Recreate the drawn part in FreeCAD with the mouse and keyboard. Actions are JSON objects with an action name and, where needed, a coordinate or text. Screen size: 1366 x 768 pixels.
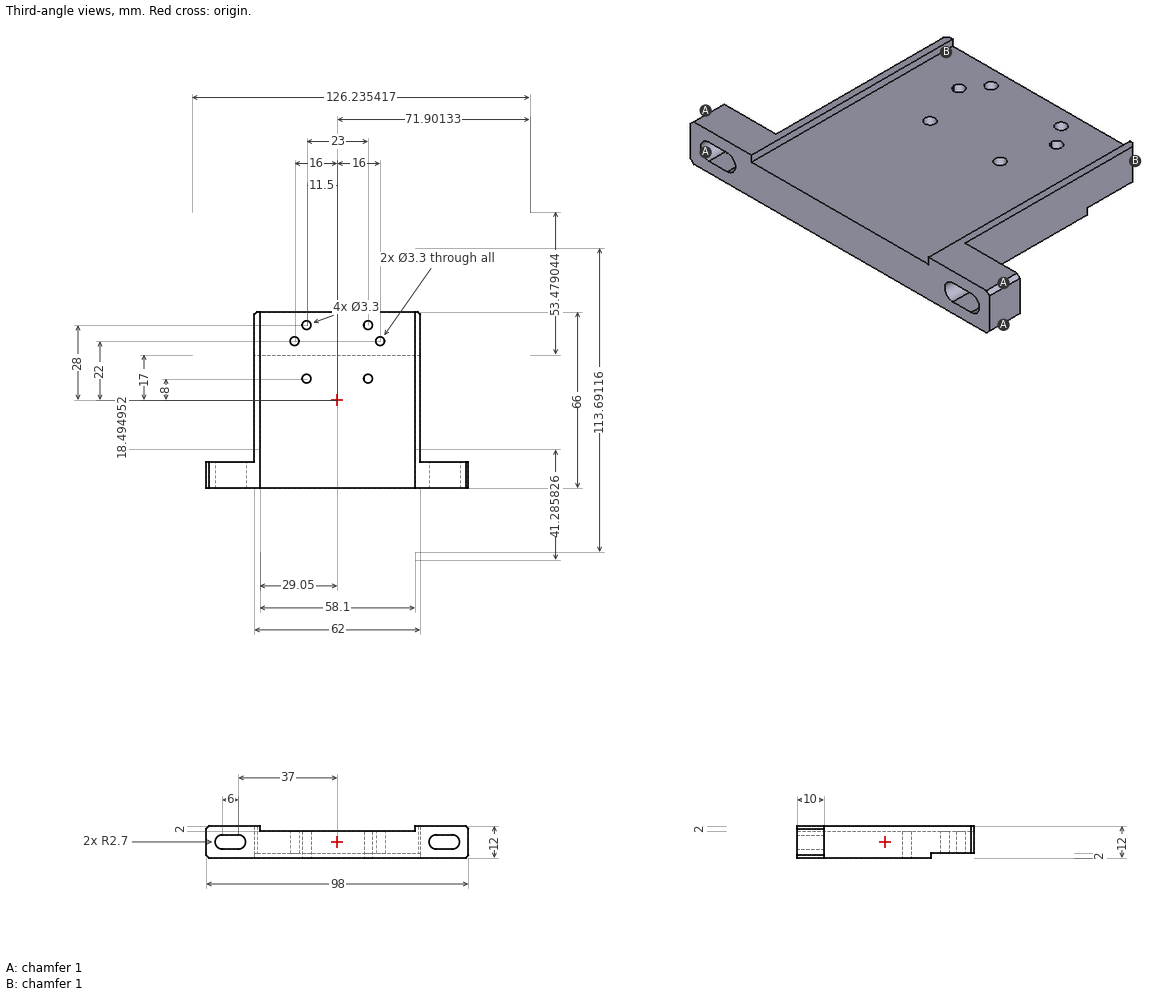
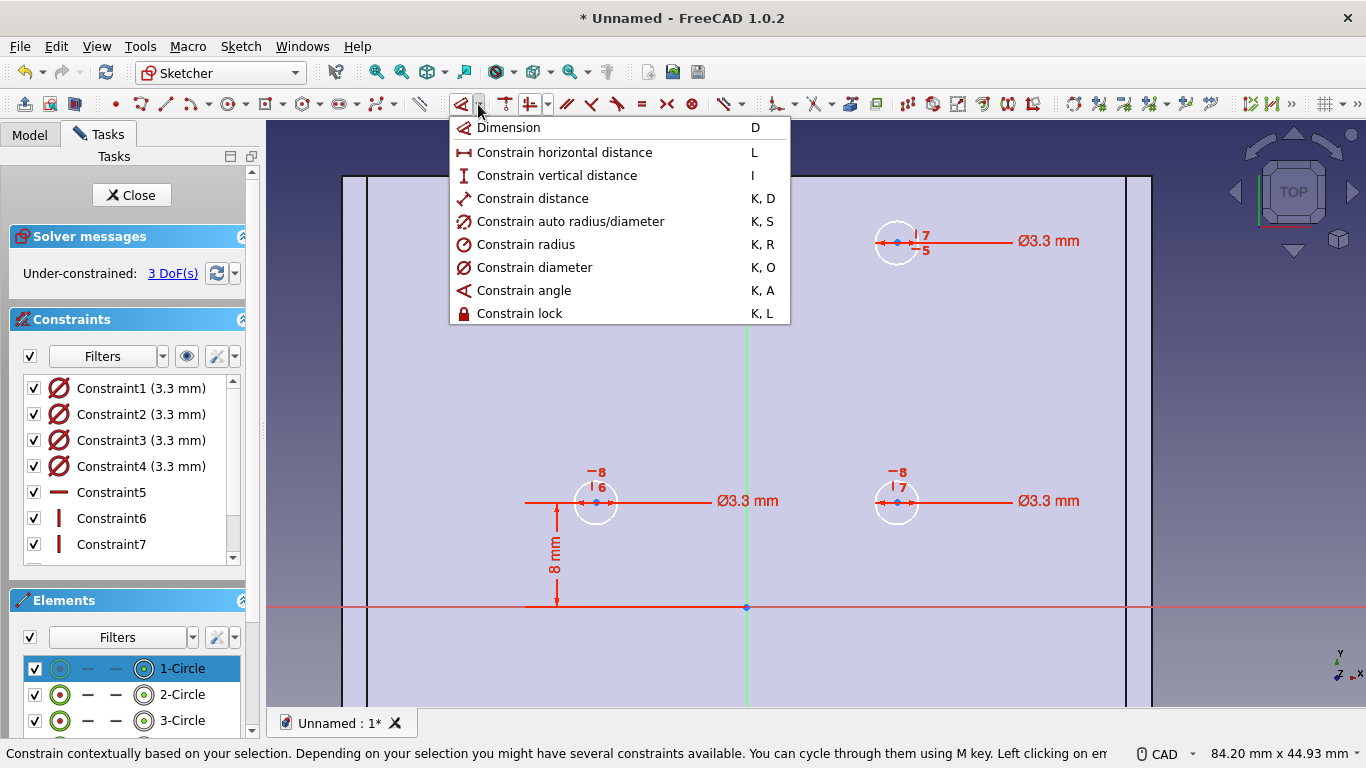
{"action": "left_click", "coordinate": [620, 176]}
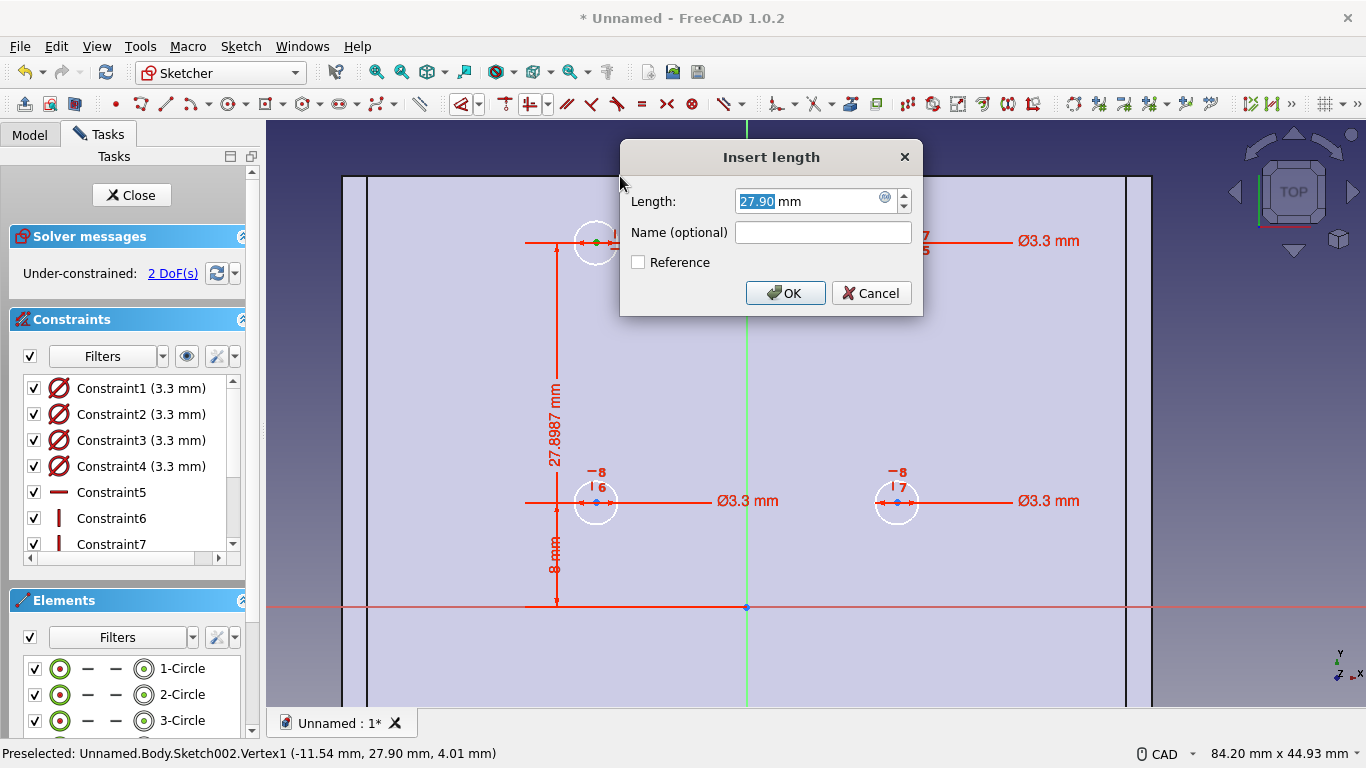
{"action": "type", "text": "28"}
{"action": "key", "text": "Return"}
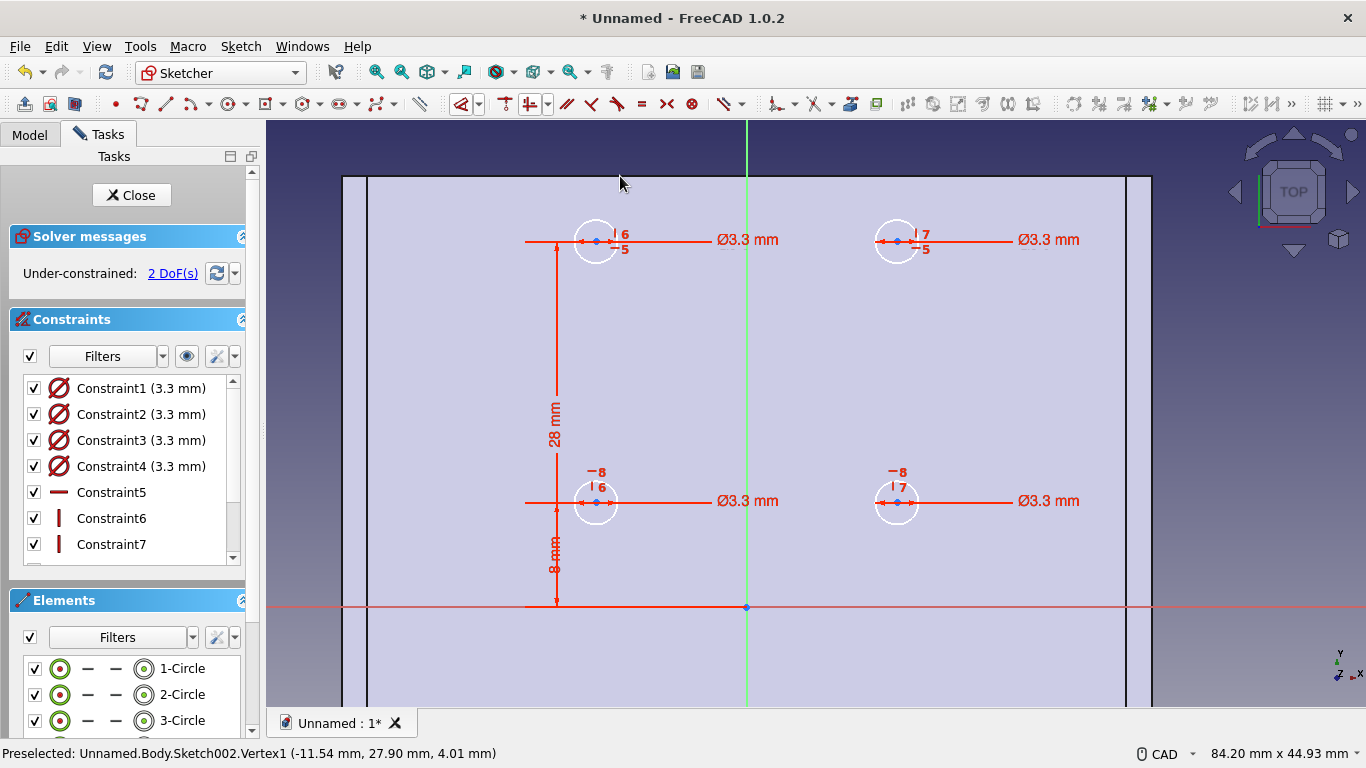
{"action": "left_click", "coordinate": [596, 242]}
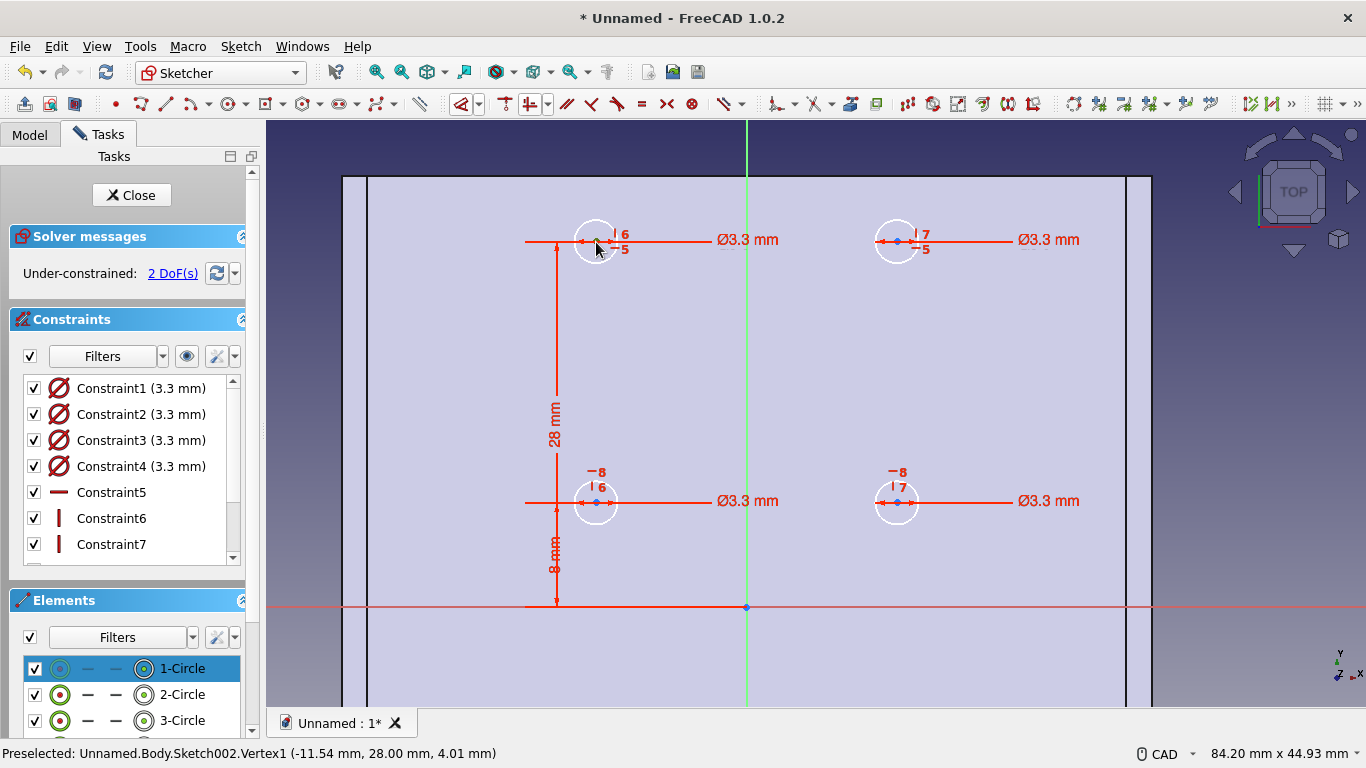
{"action": "left_click", "coordinate": [897, 242]}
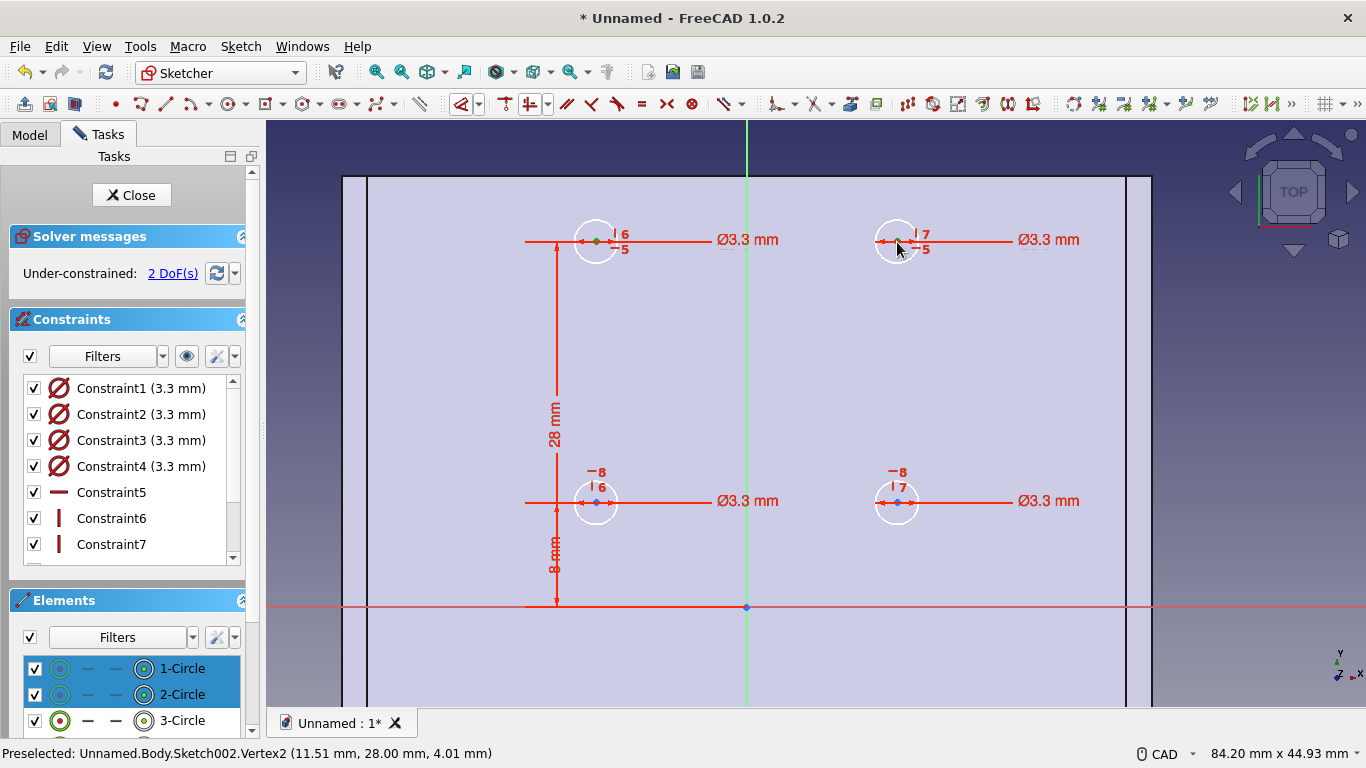
{"action": "key", "text": "l"}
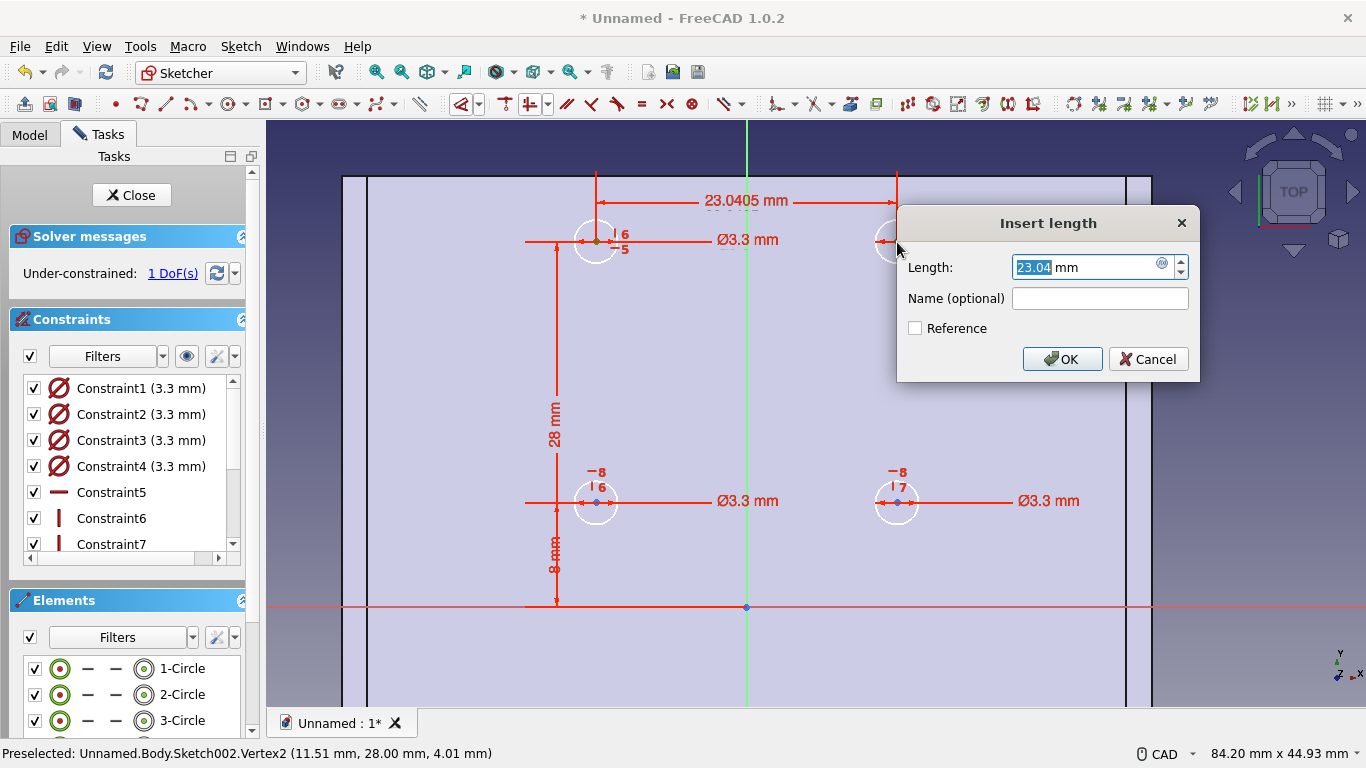
{"action": "type", "text": "23"}
{"action": "key", "text": "Return"}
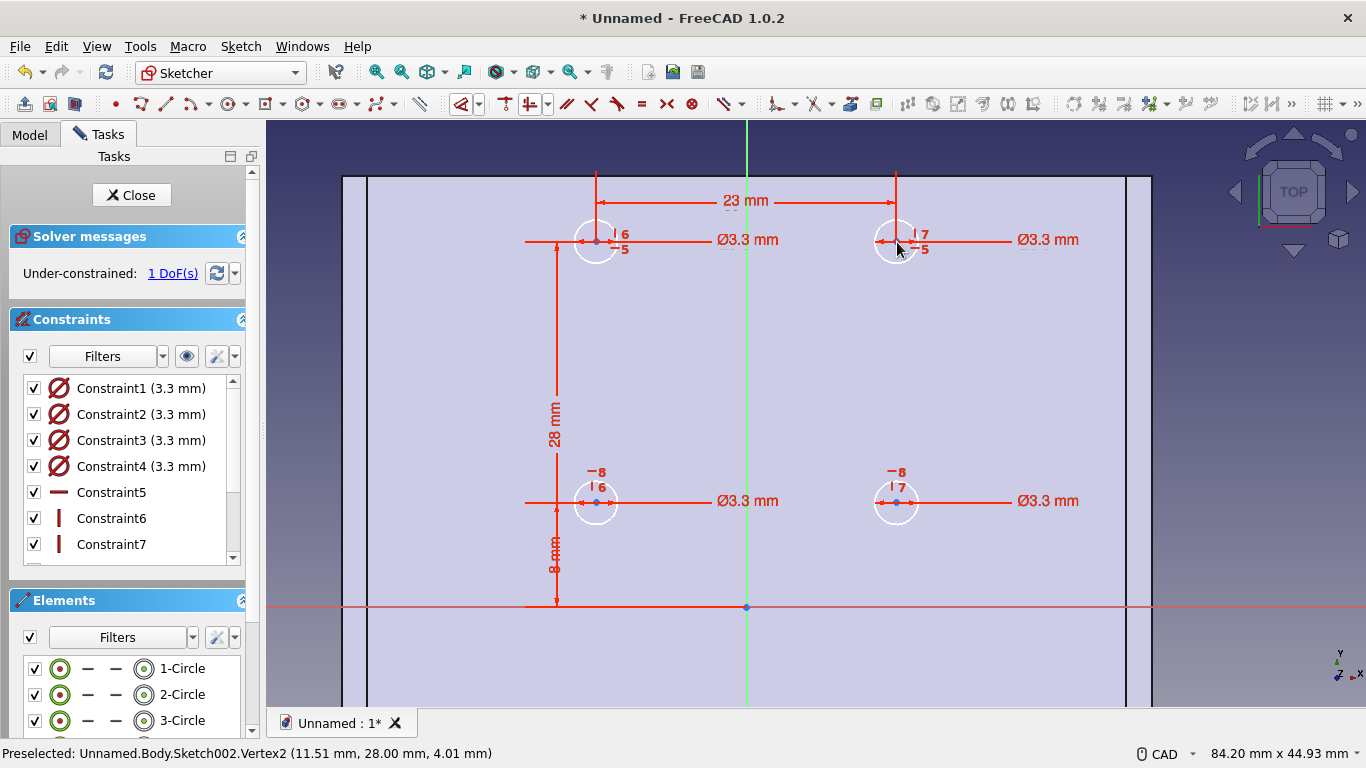
{"action": "left_click", "coordinate": [596, 242]}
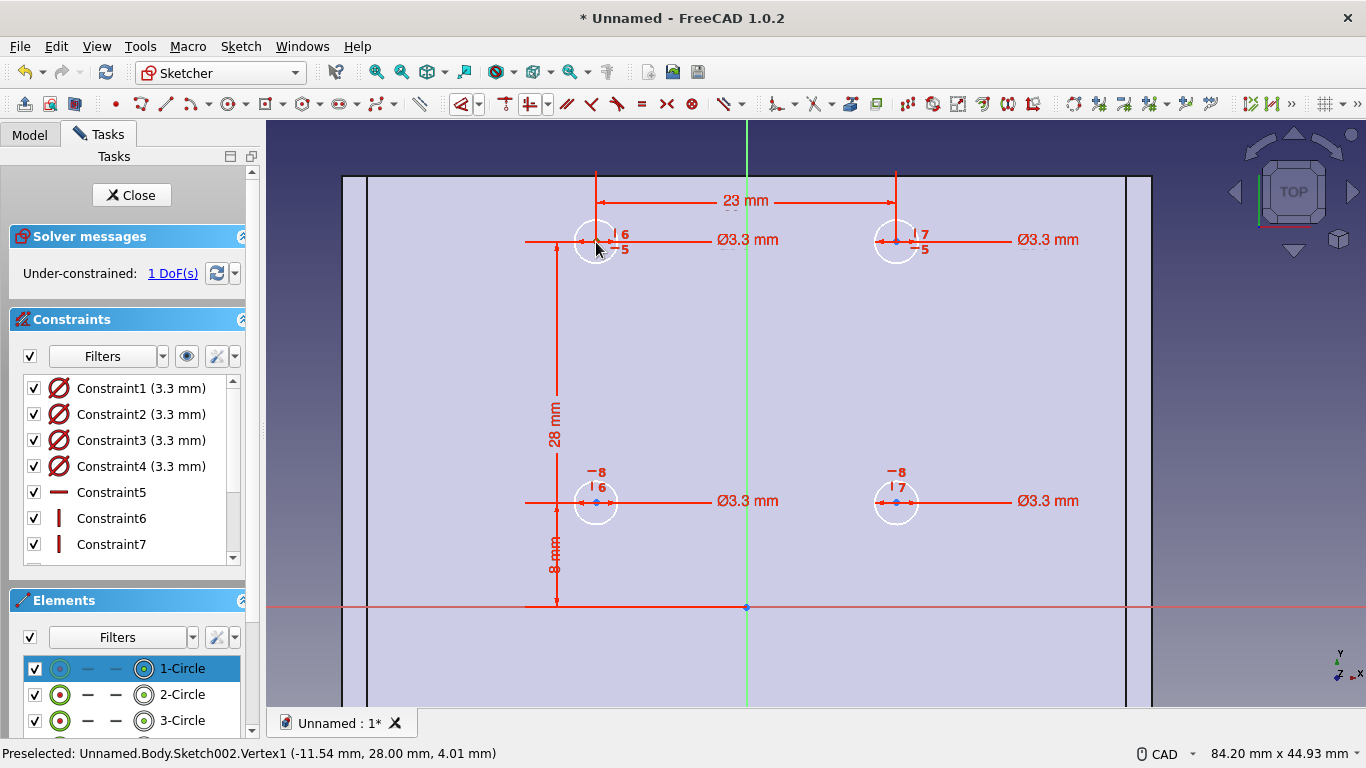
{"action": "left_click", "coordinate": [478, 104]}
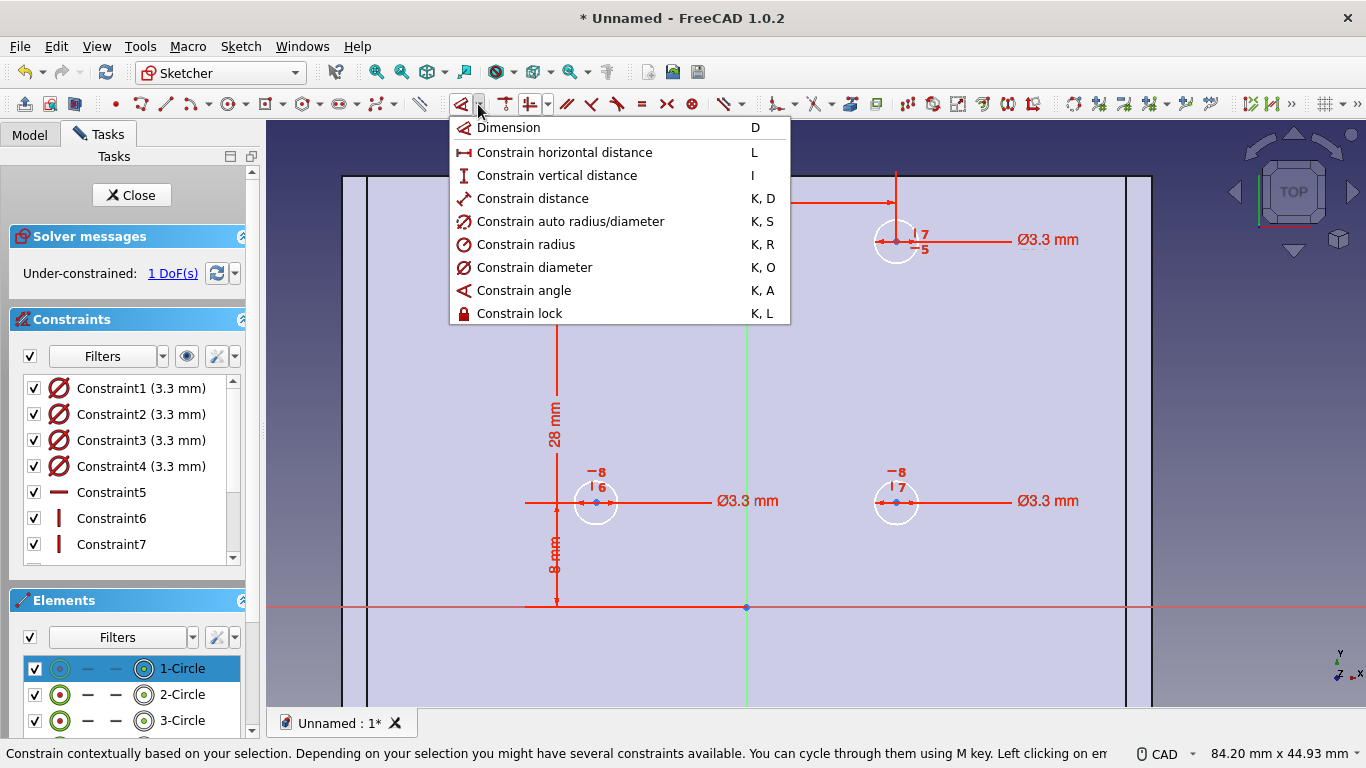
{"action": "left_click", "coordinate": [620, 152]}